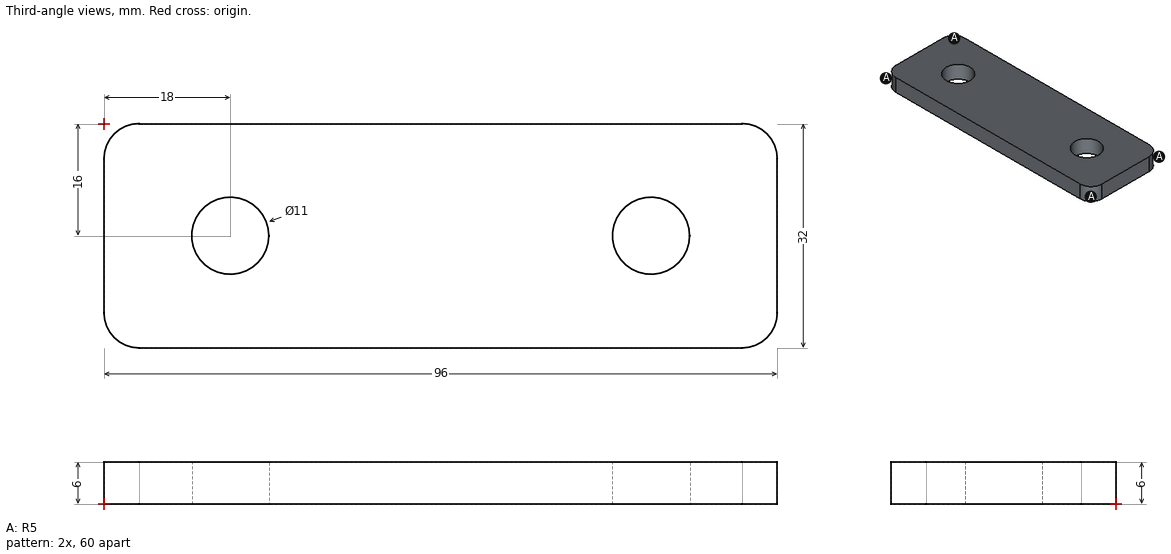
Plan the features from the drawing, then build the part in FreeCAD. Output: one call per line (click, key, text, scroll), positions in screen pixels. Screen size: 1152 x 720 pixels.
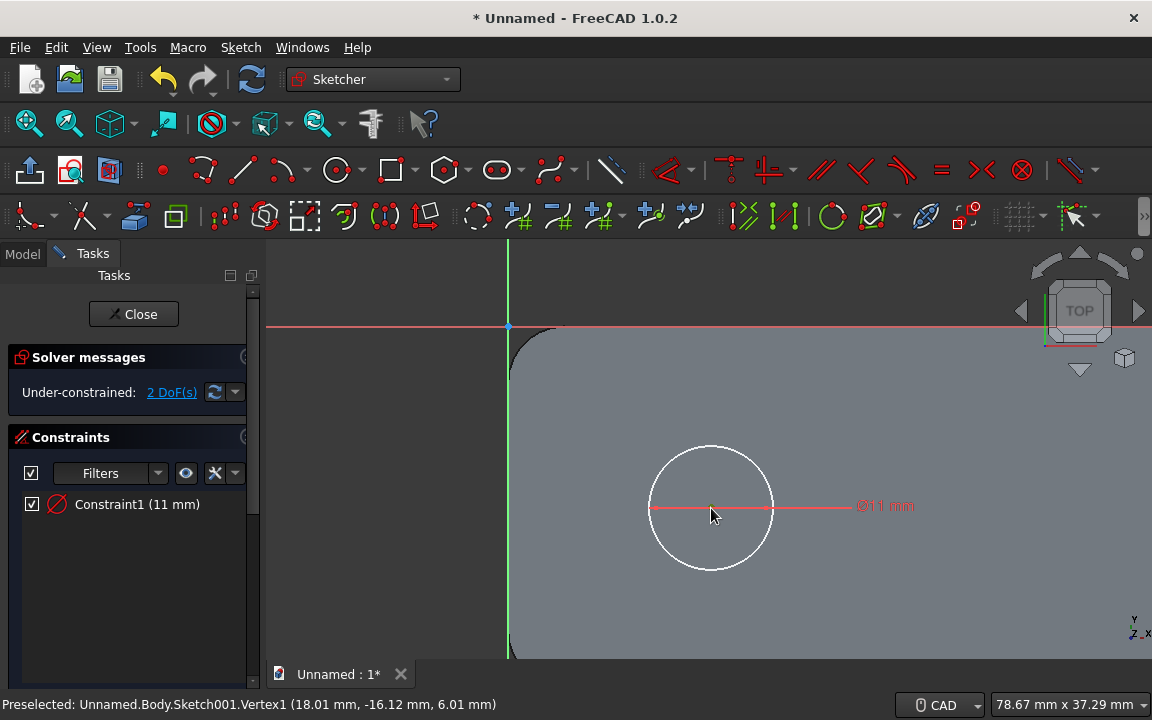
key(l)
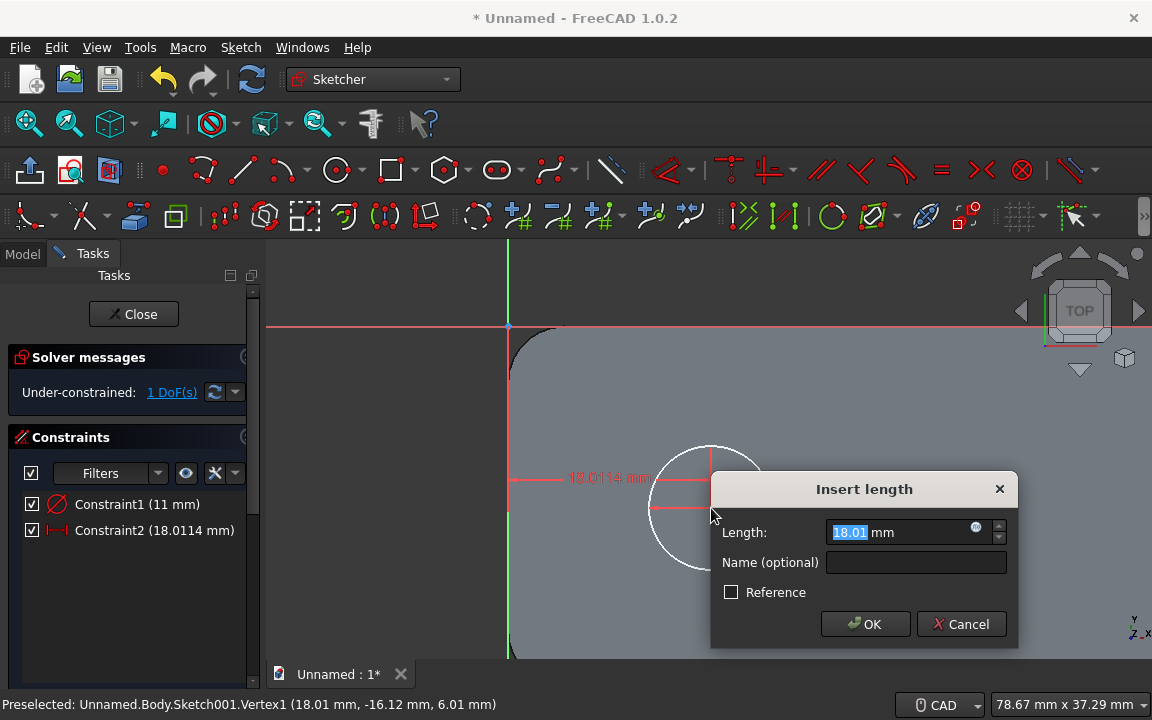
text(18)
key(Return)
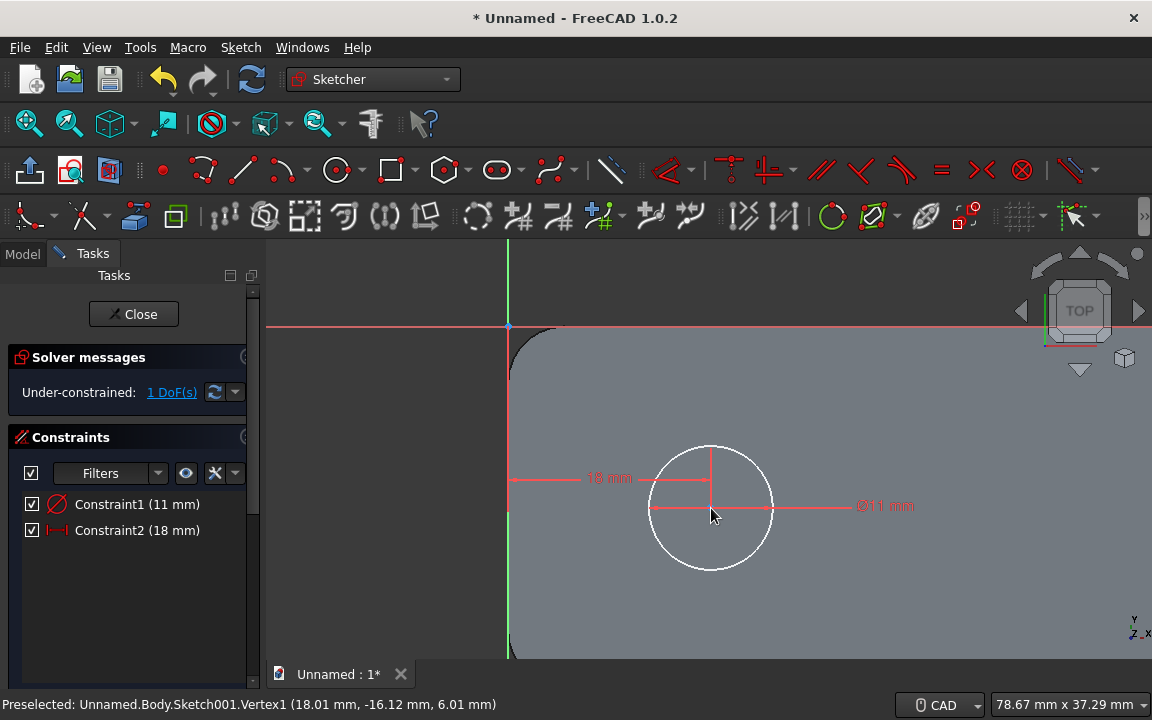
click(711, 508)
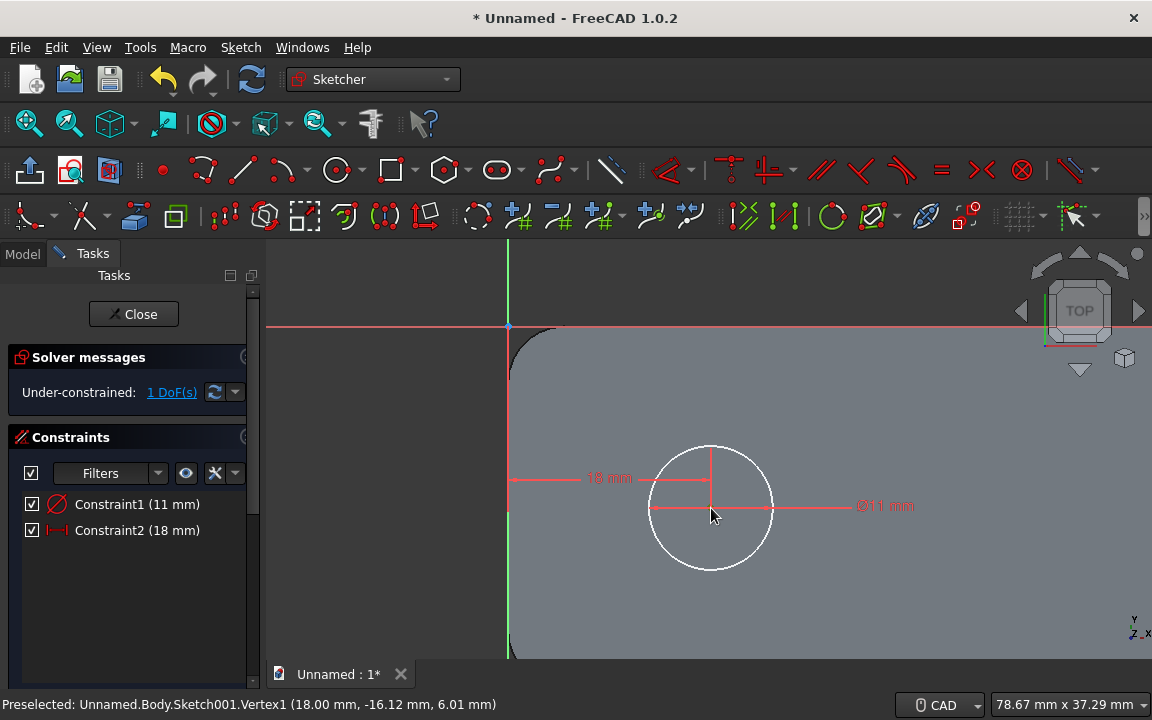
key(i)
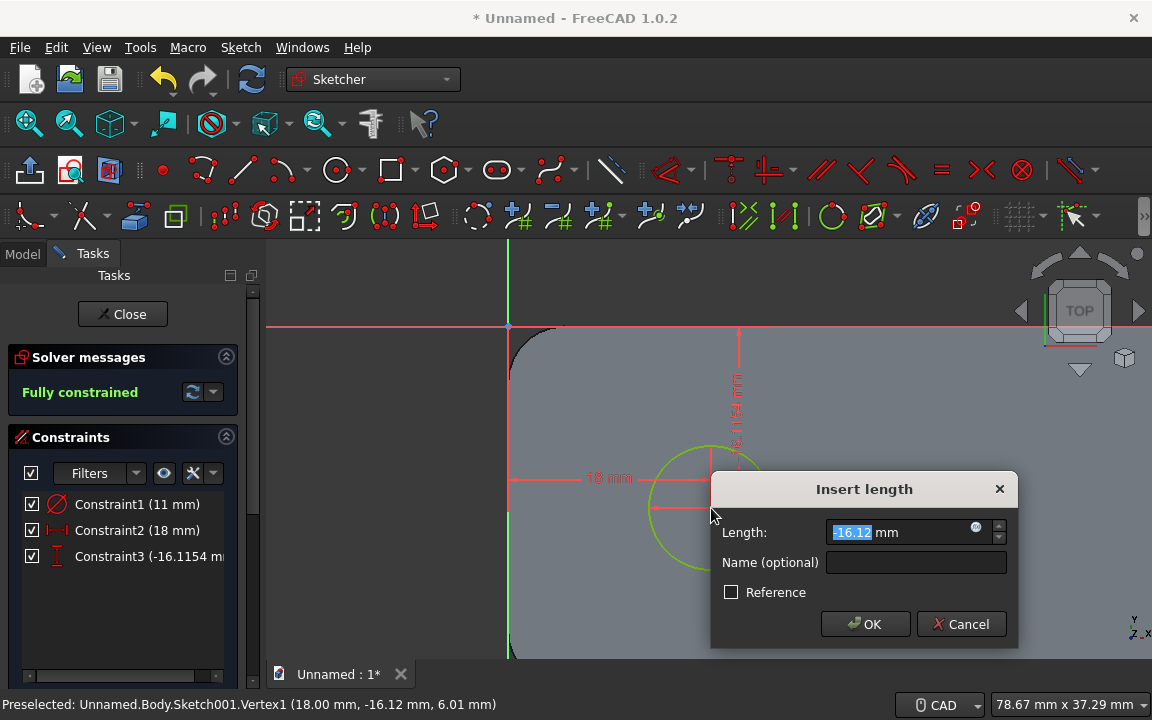
text(-16)
key(Return)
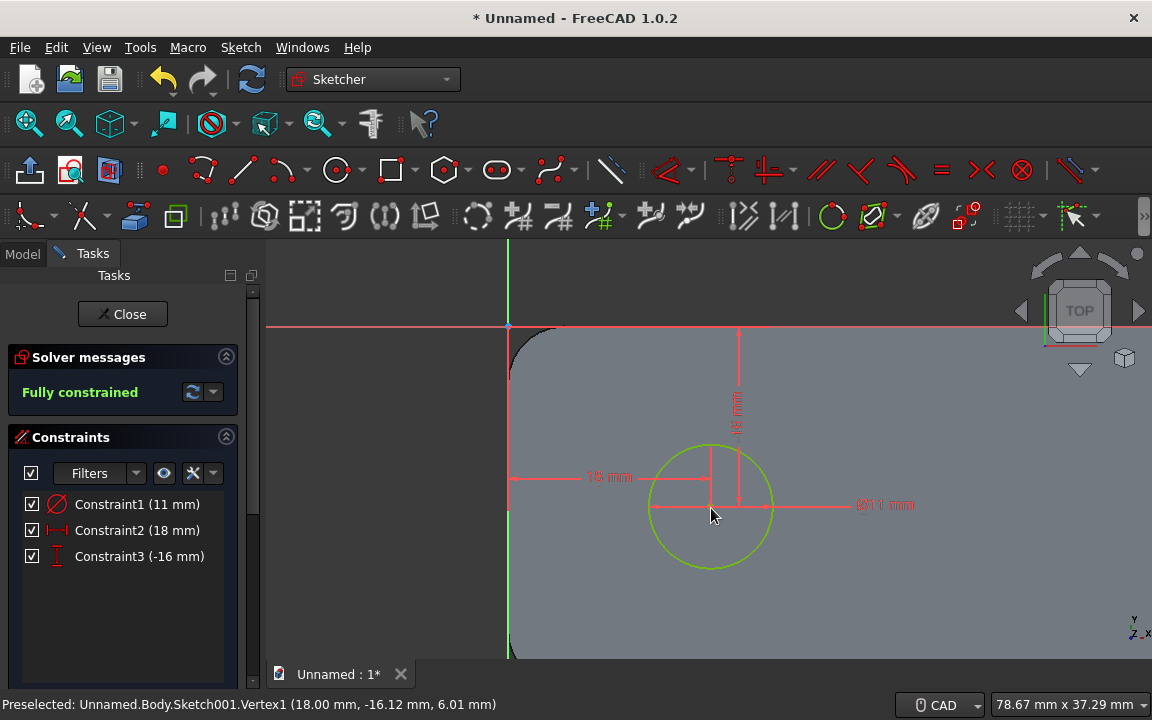
click(123, 314)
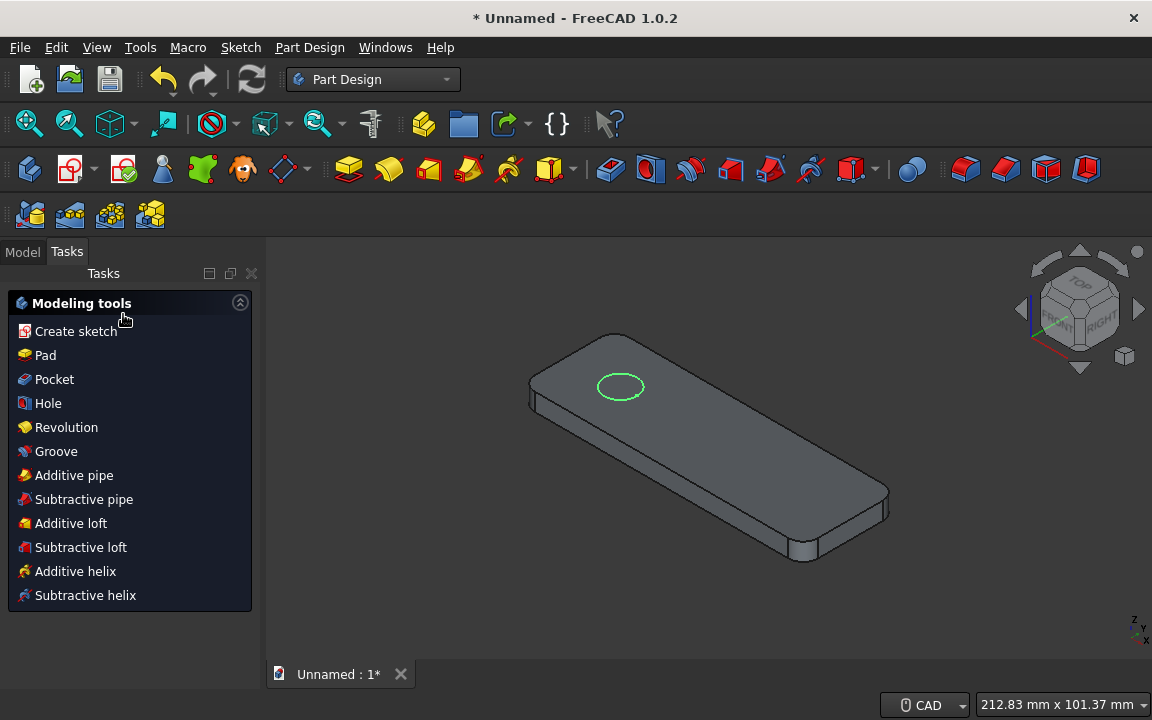
click(612, 170)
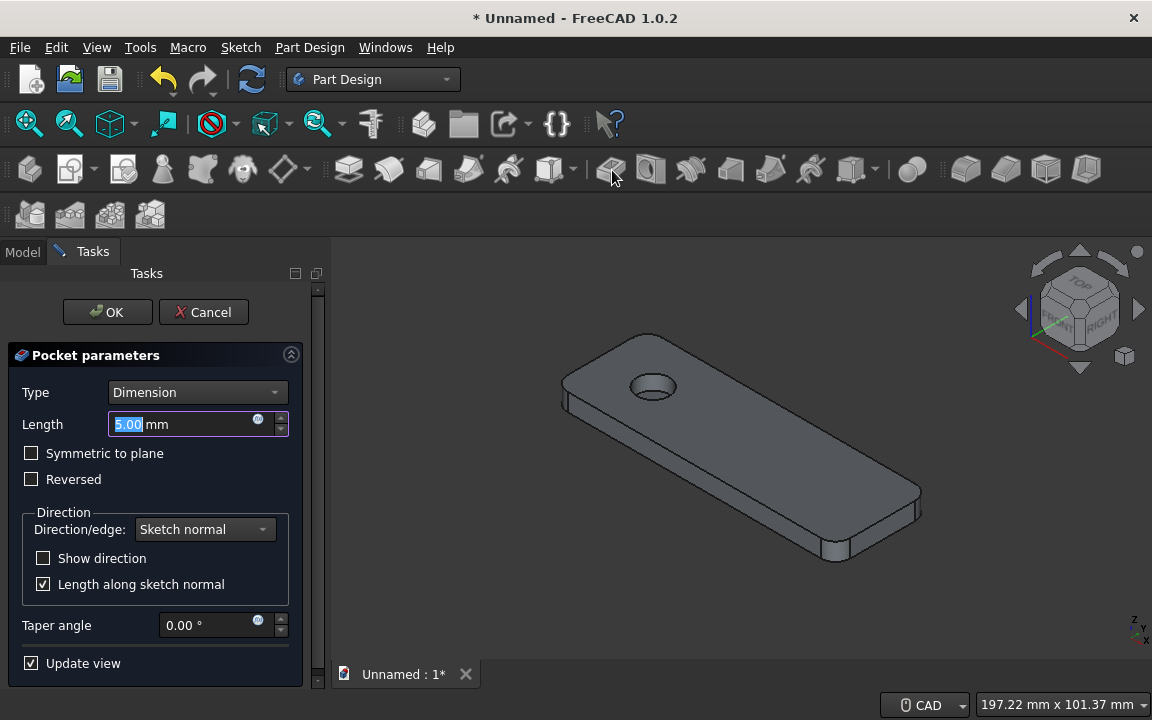
text(6)
key(Tab)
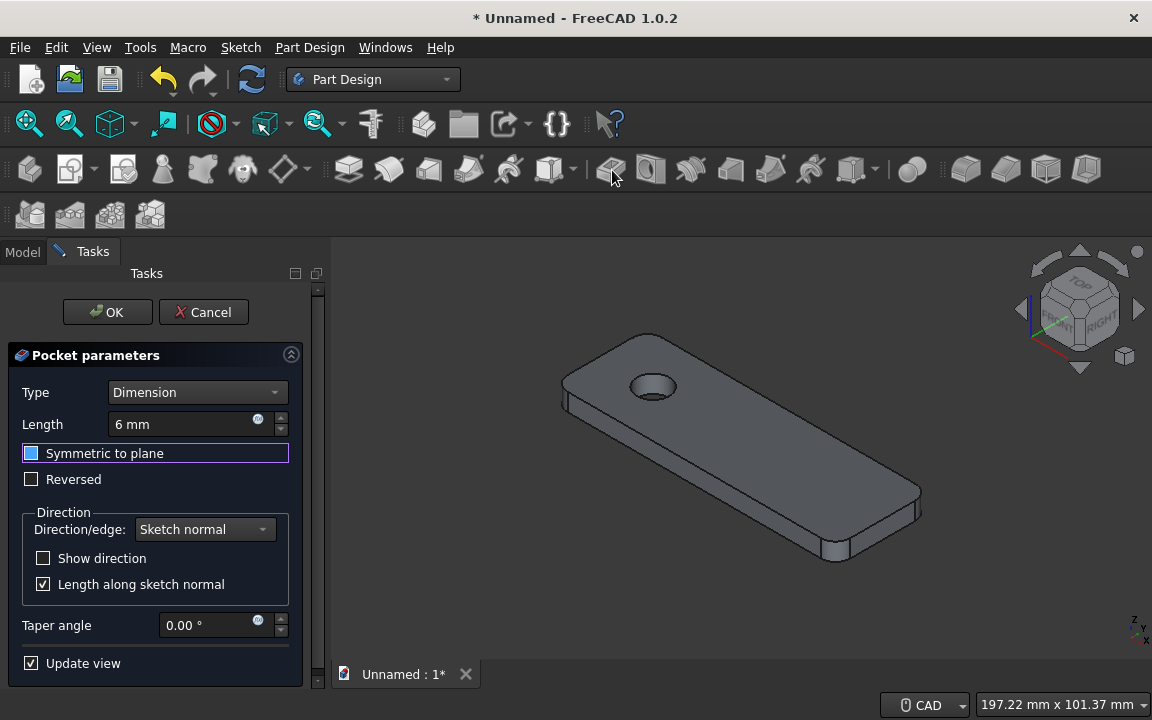
click(108, 312)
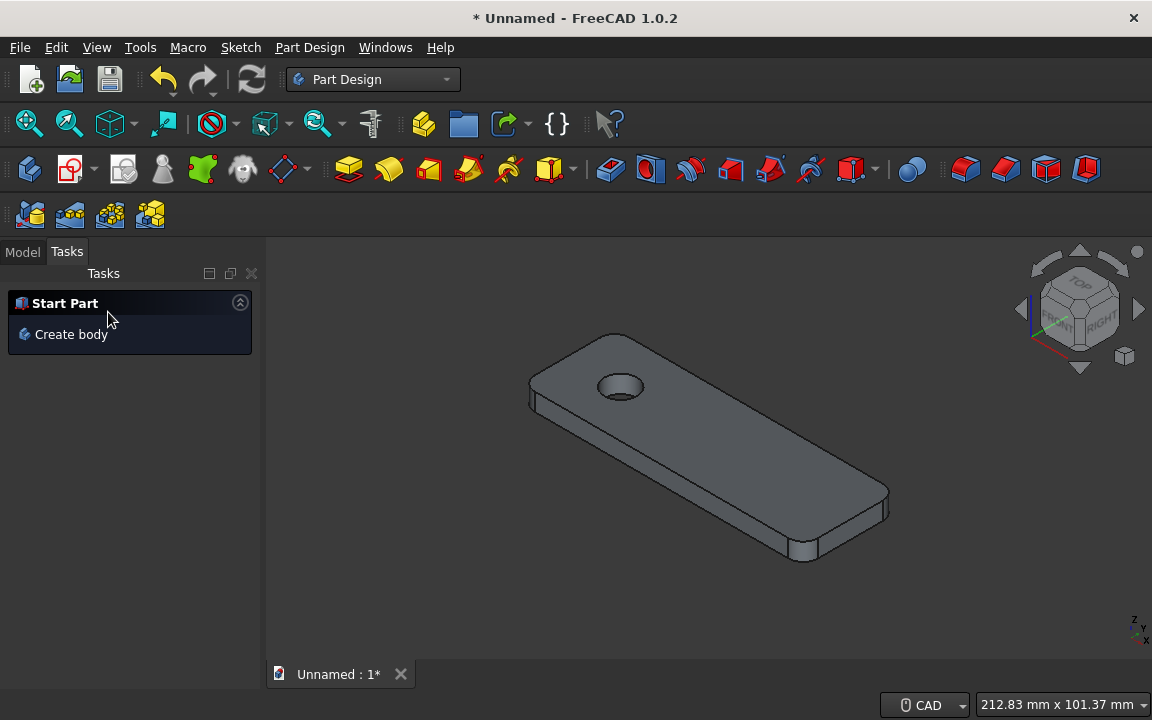
click(23, 251)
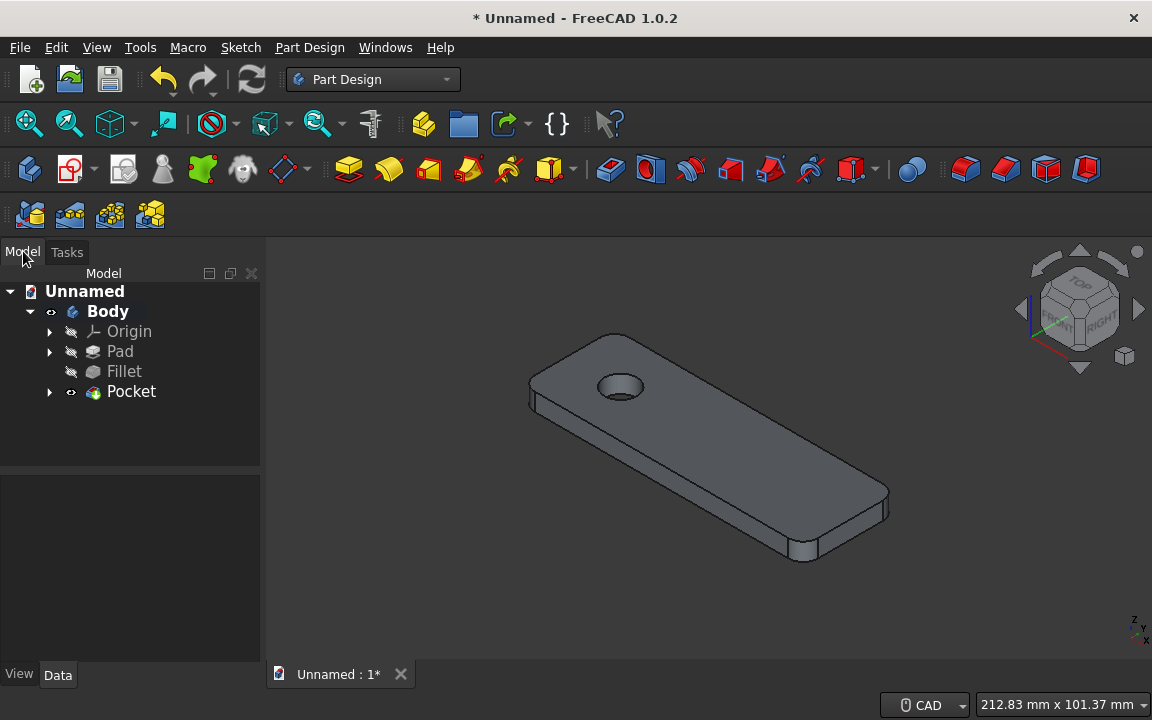
click(116, 392)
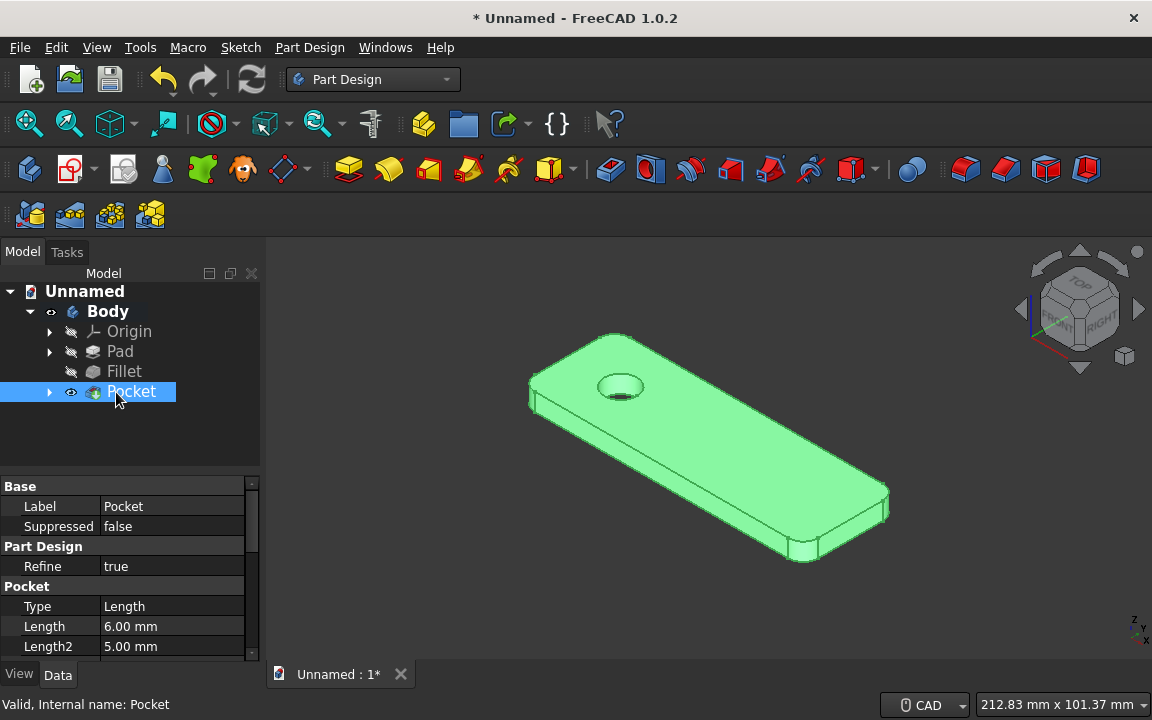
click(70, 214)